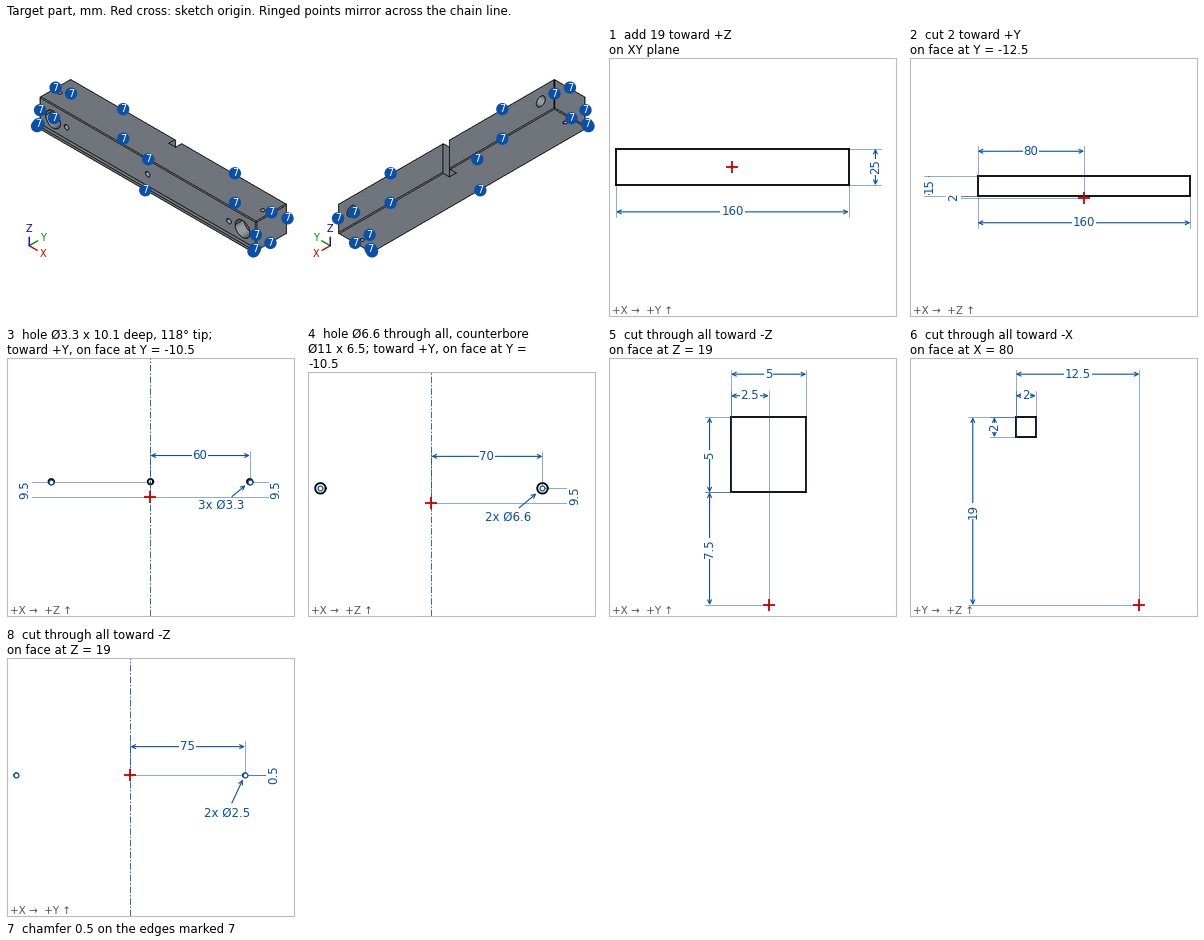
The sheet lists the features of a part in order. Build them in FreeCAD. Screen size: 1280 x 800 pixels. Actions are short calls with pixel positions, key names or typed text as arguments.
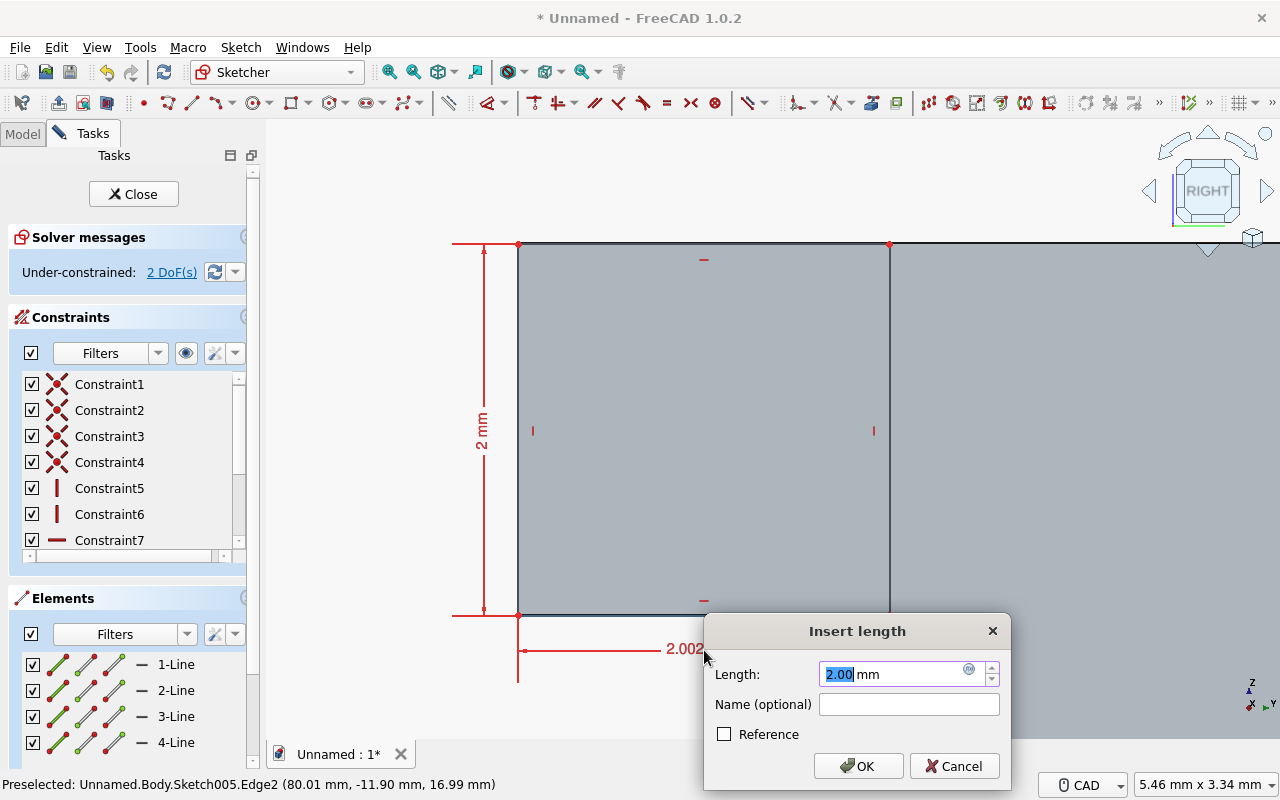
text(2)
key(Return)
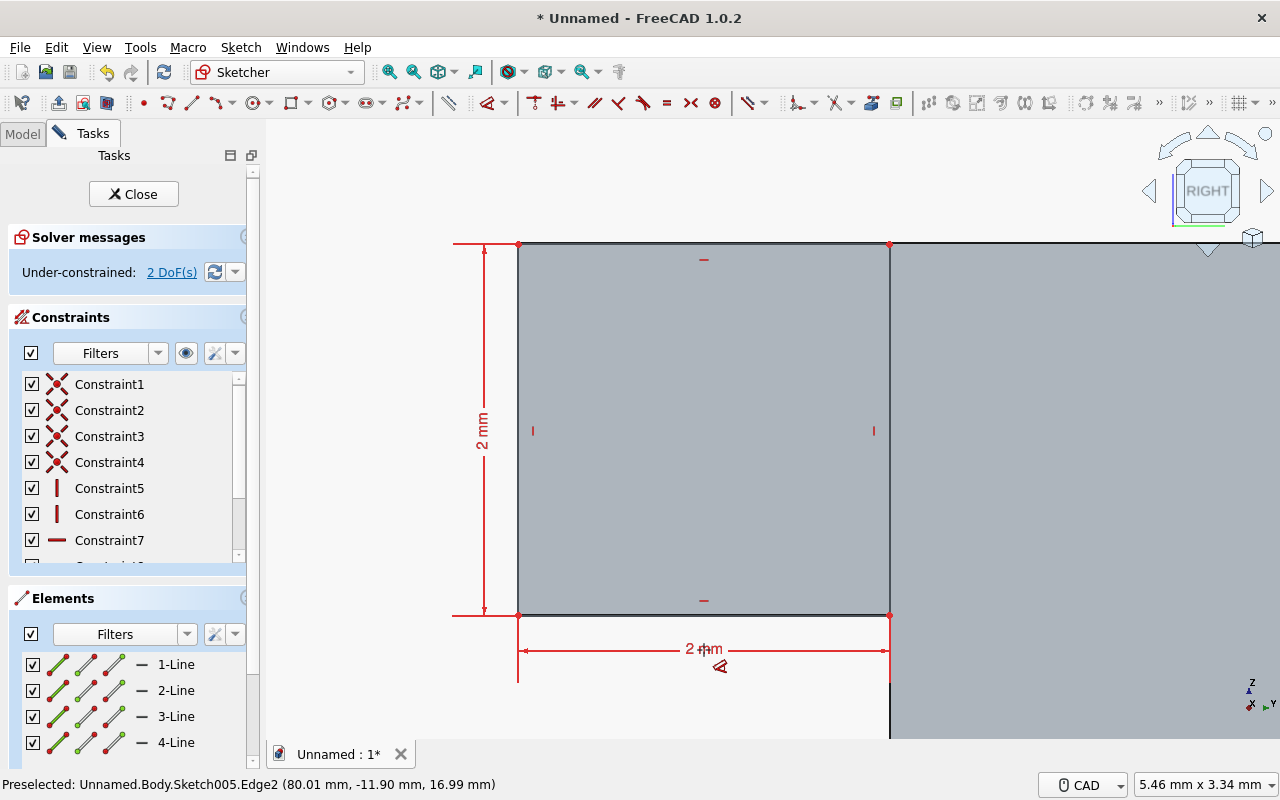
click(518, 244)
click(484, 478)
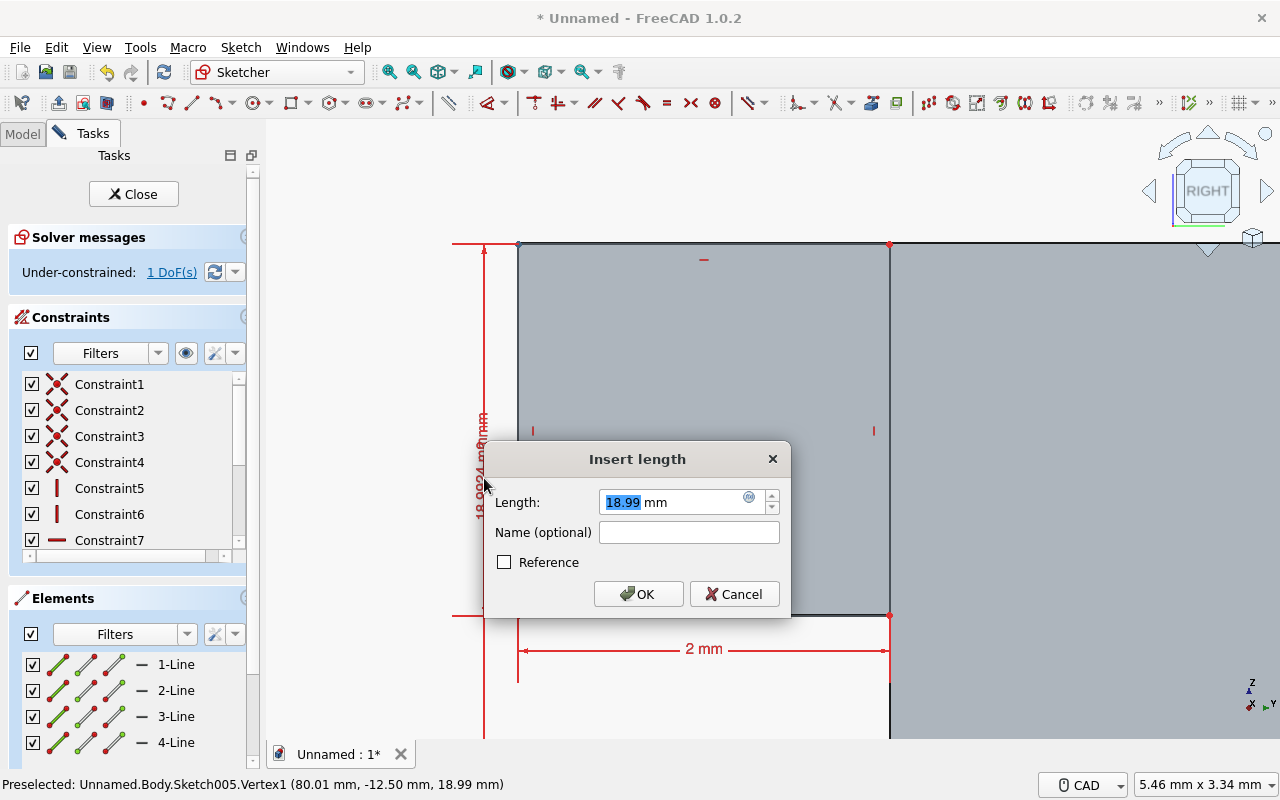
text(19)
key(Return)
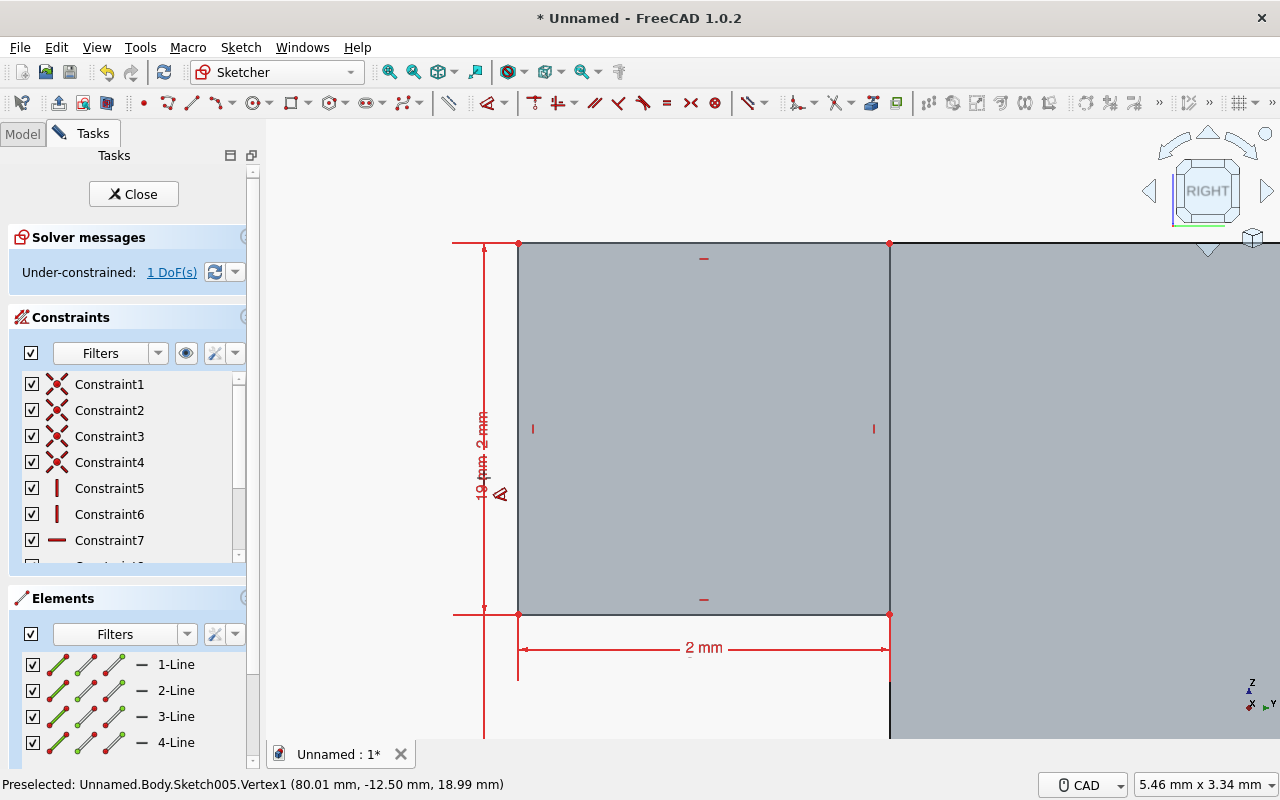
click(518, 243)
click(817, 209)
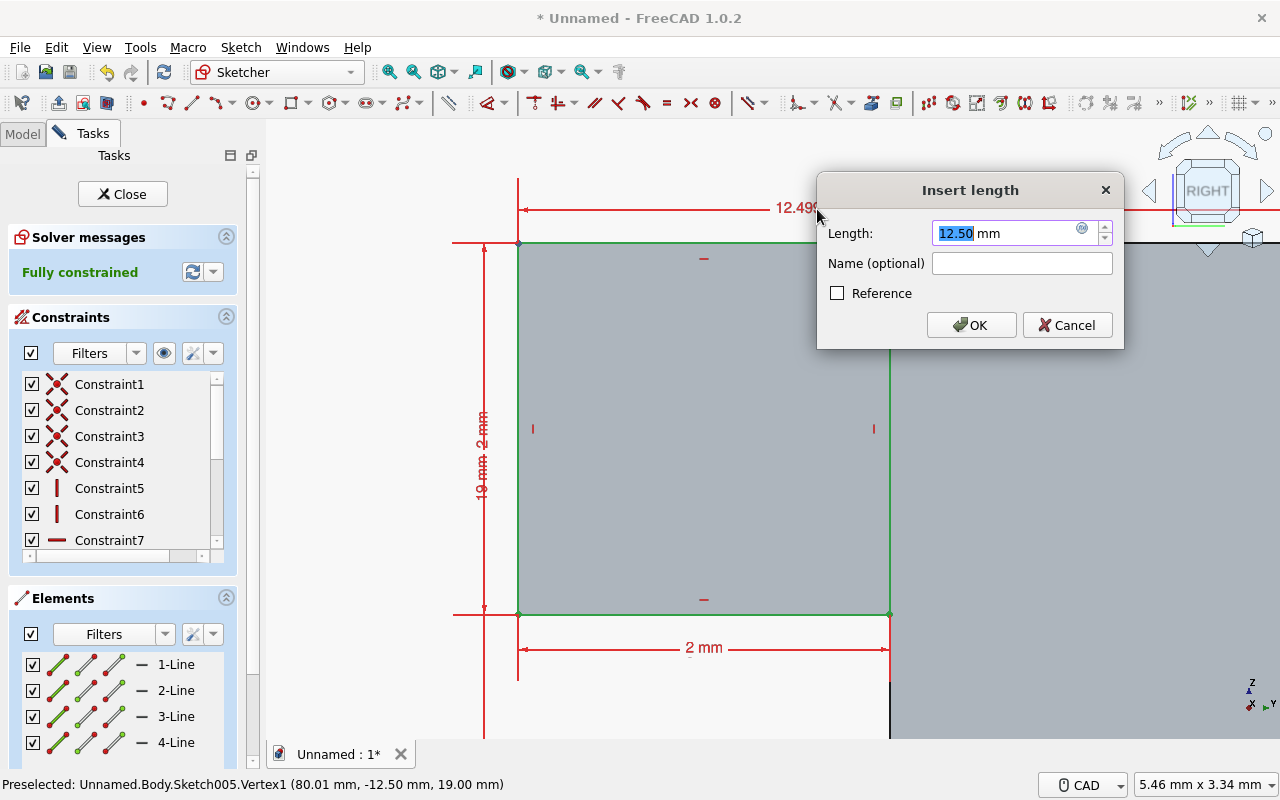
text(12.5)
key(Return)
key(Escape)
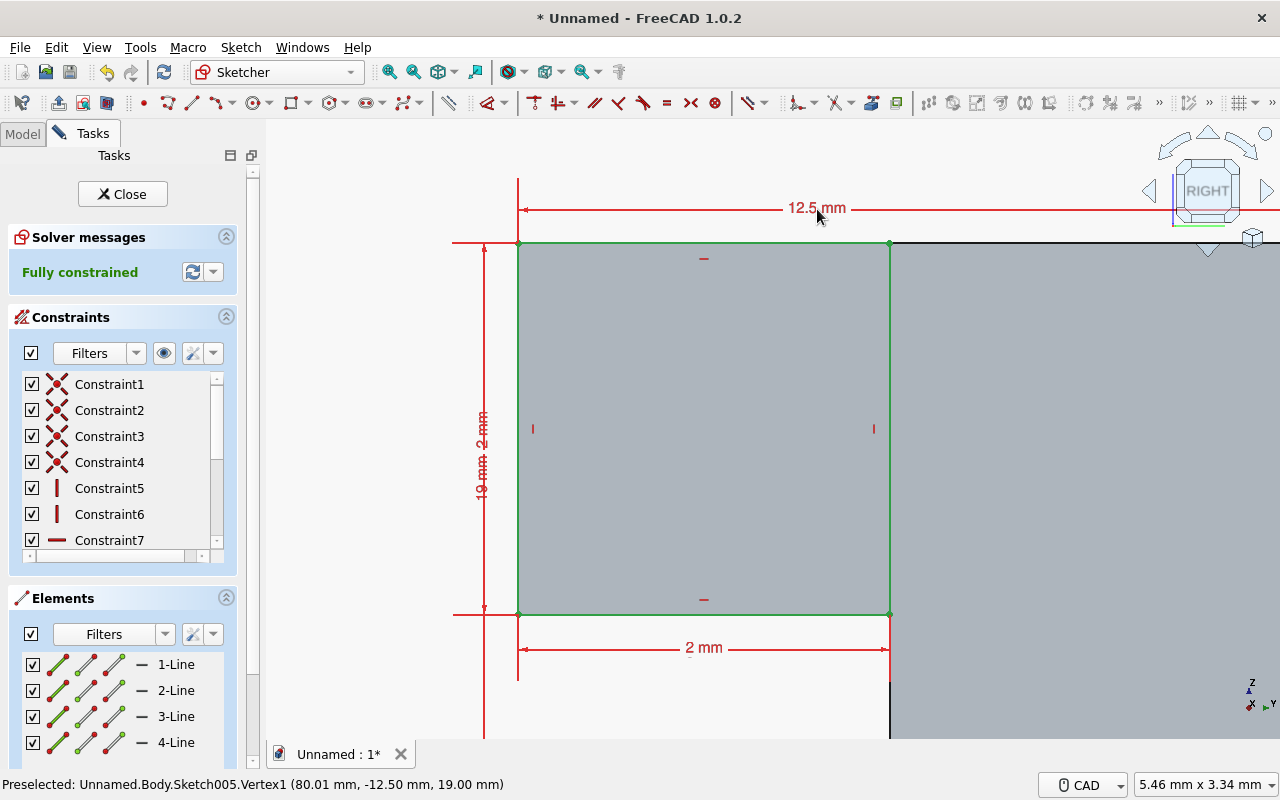
click(123, 194)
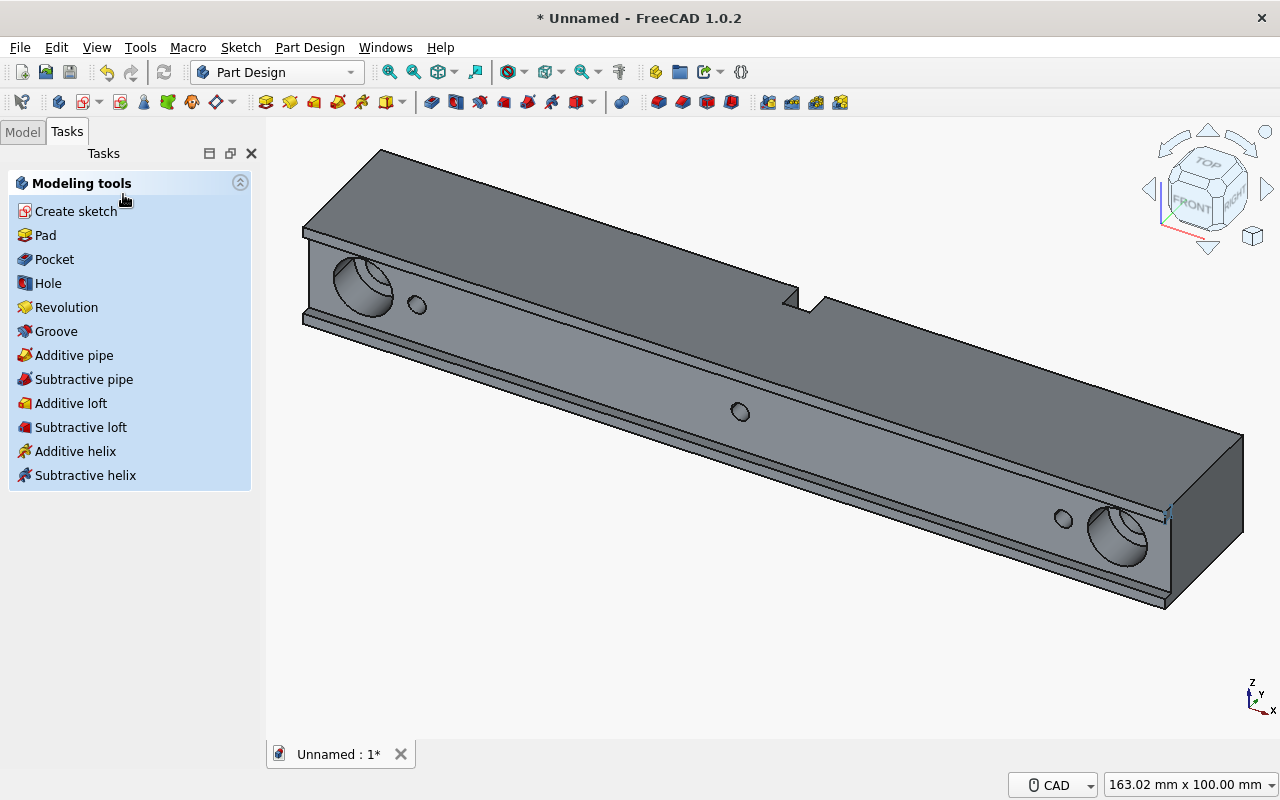
click(432, 102)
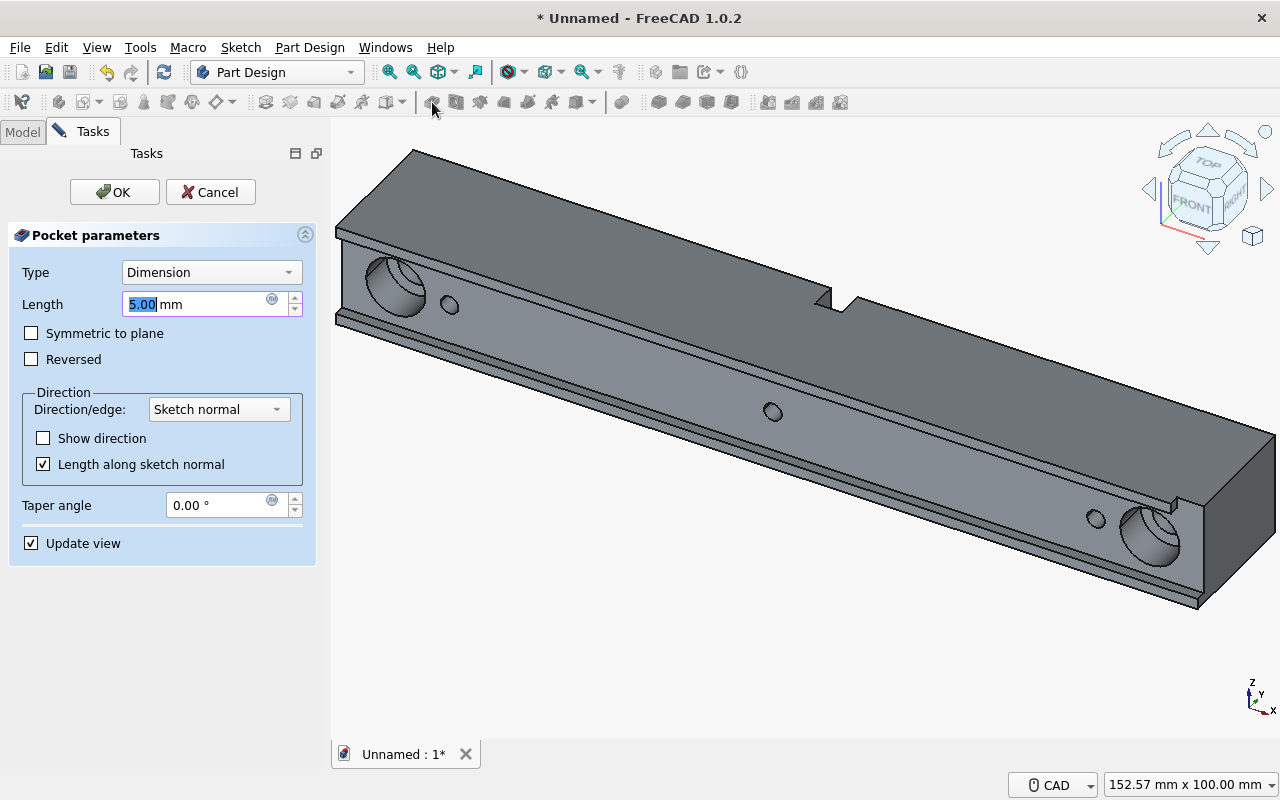
click(212, 272)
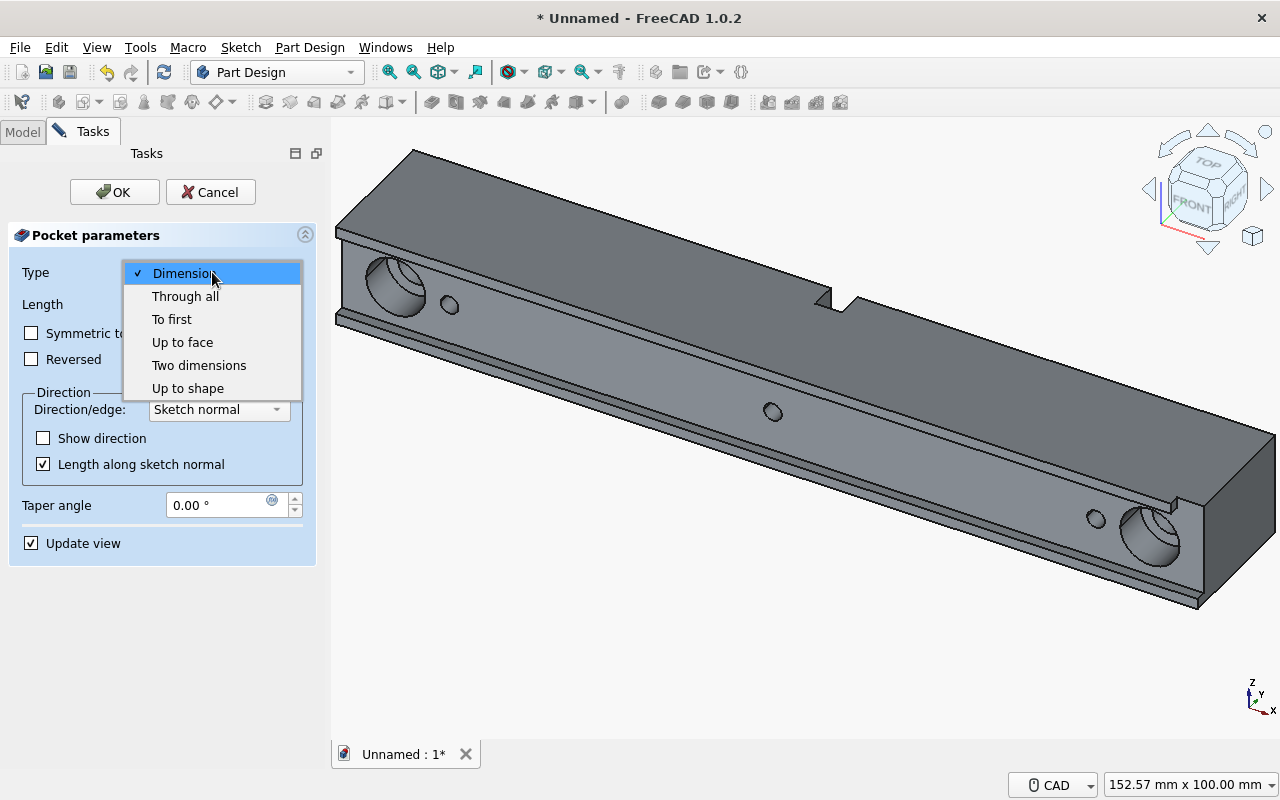
click(212, 296)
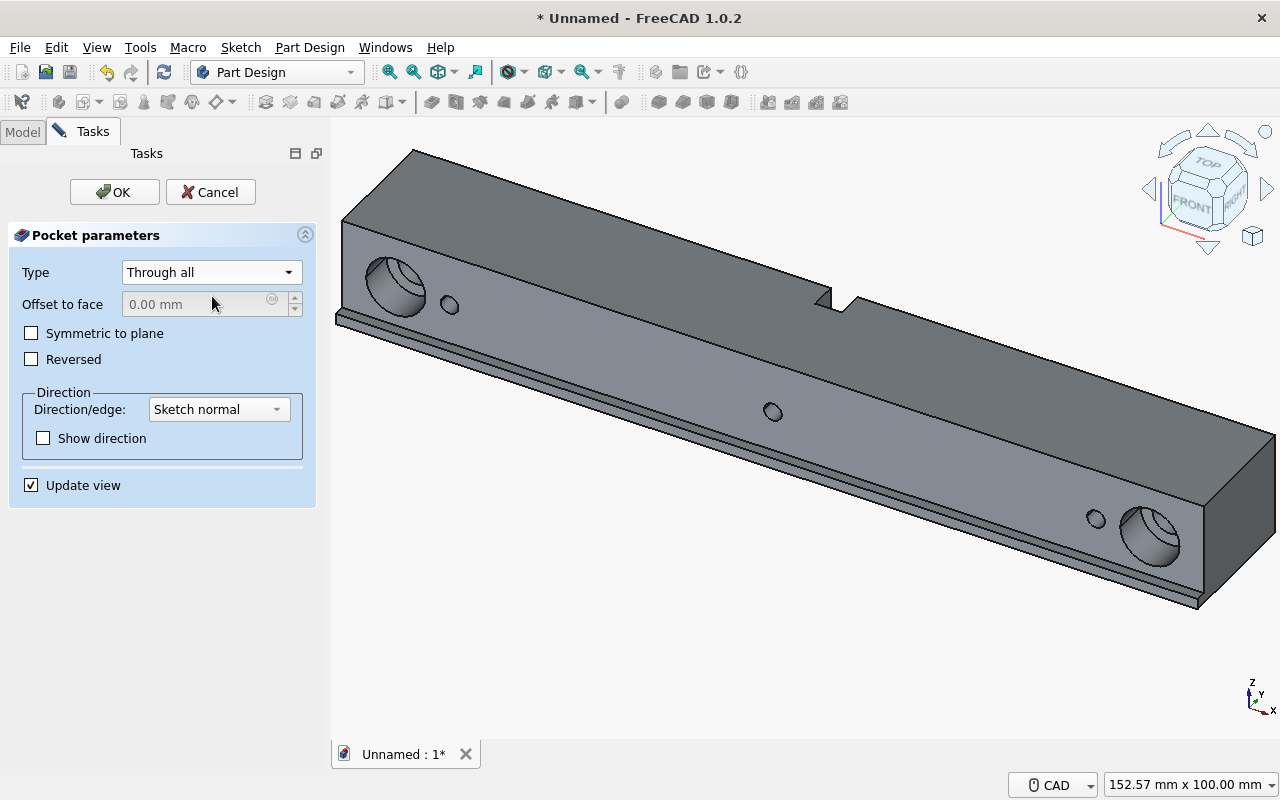
click(115, 192)